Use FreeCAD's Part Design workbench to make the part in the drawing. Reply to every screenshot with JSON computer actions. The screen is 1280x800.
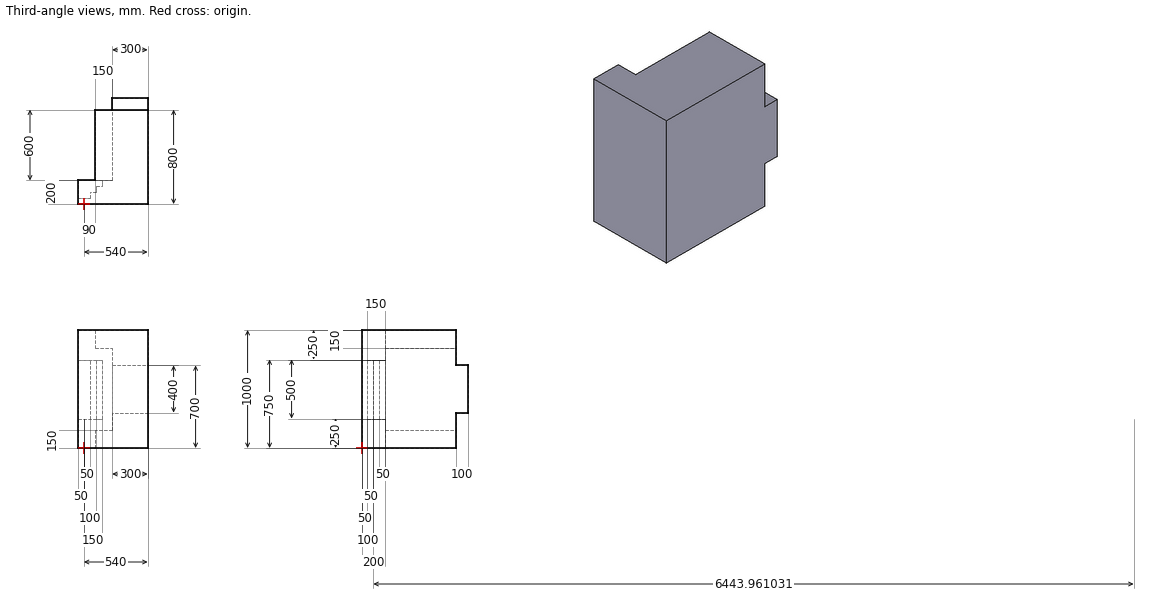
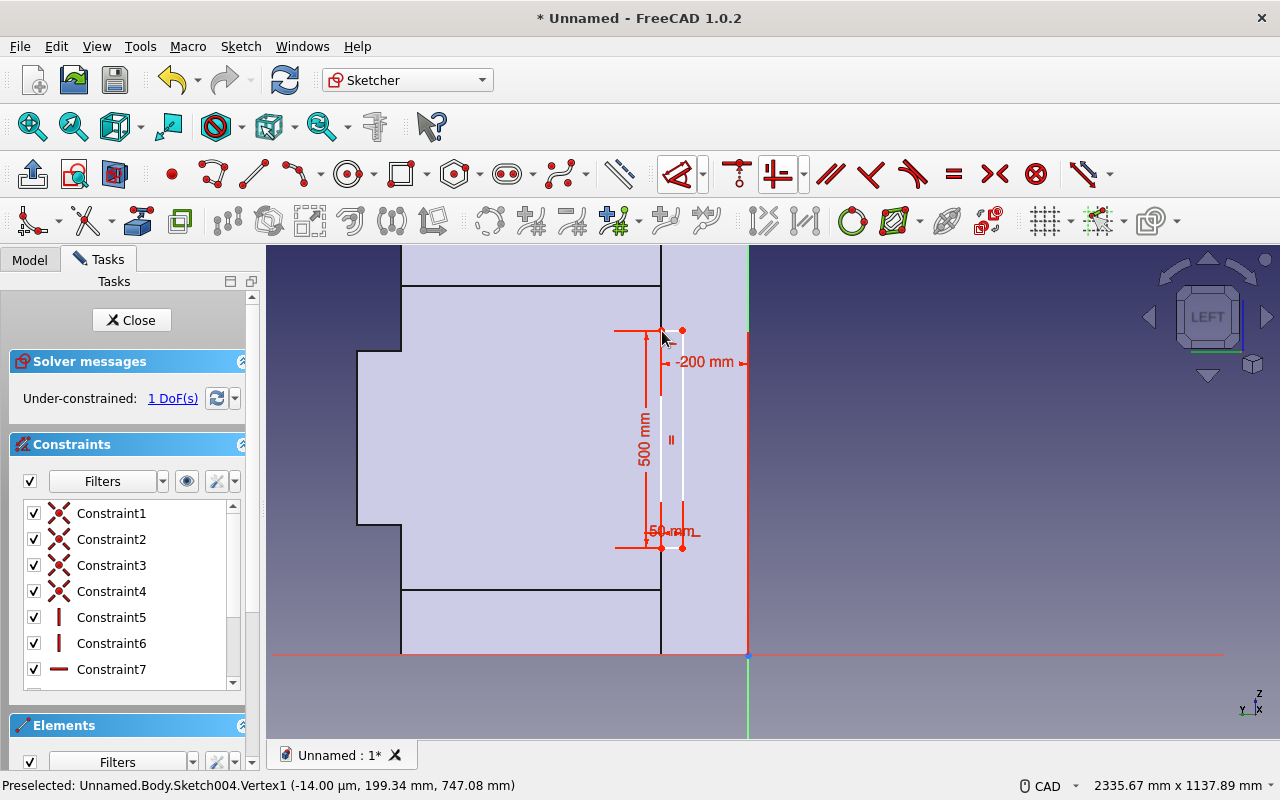
{"action": "left_click", "coordinate": [661, 331]}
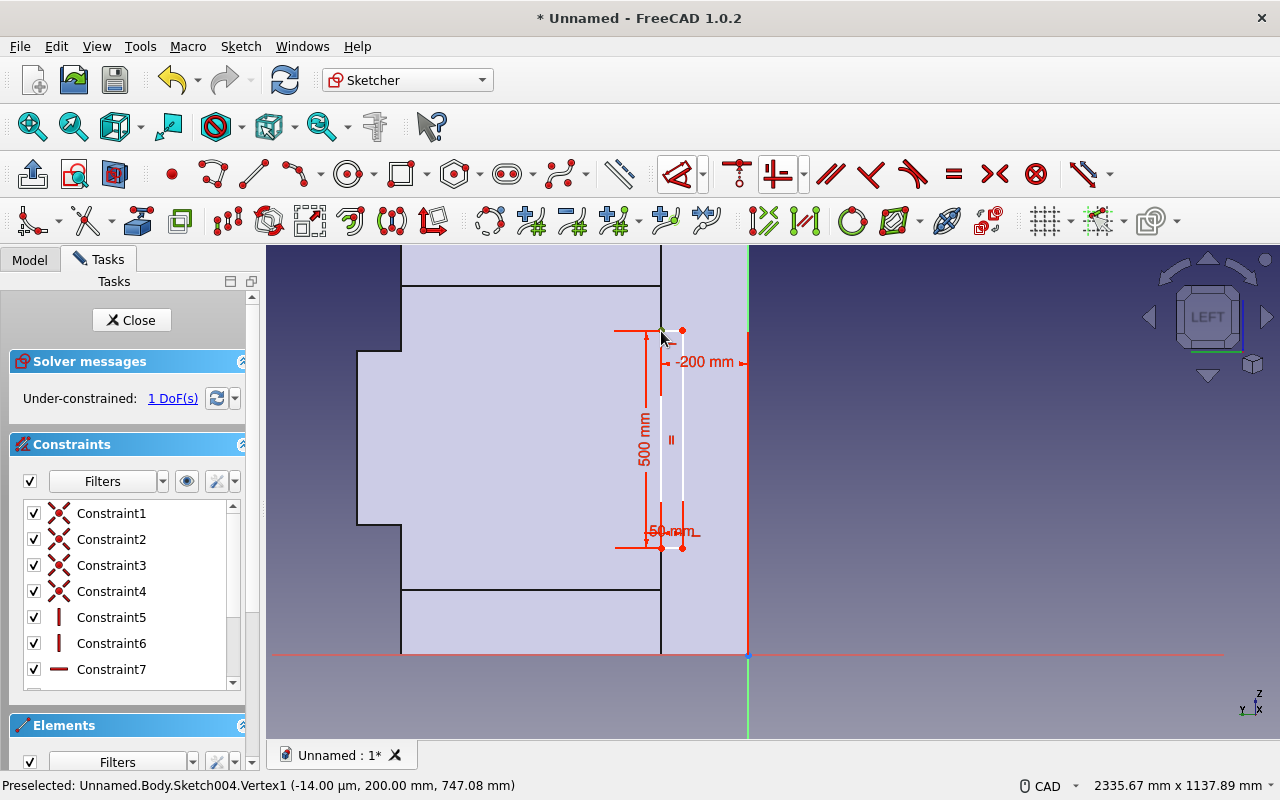
{"action": "key", "text": "i"}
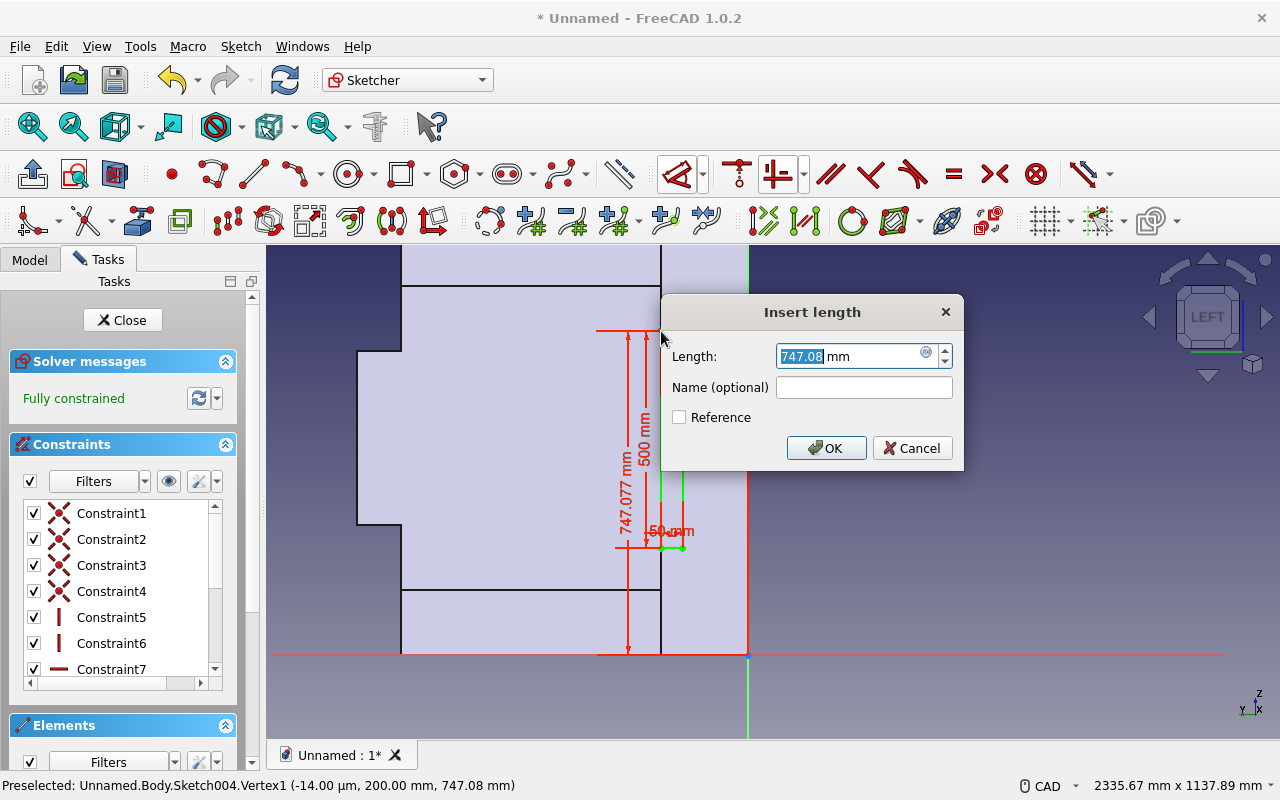
{"action": "type", "text": "750"}
{"action": "key", "text": "Return"}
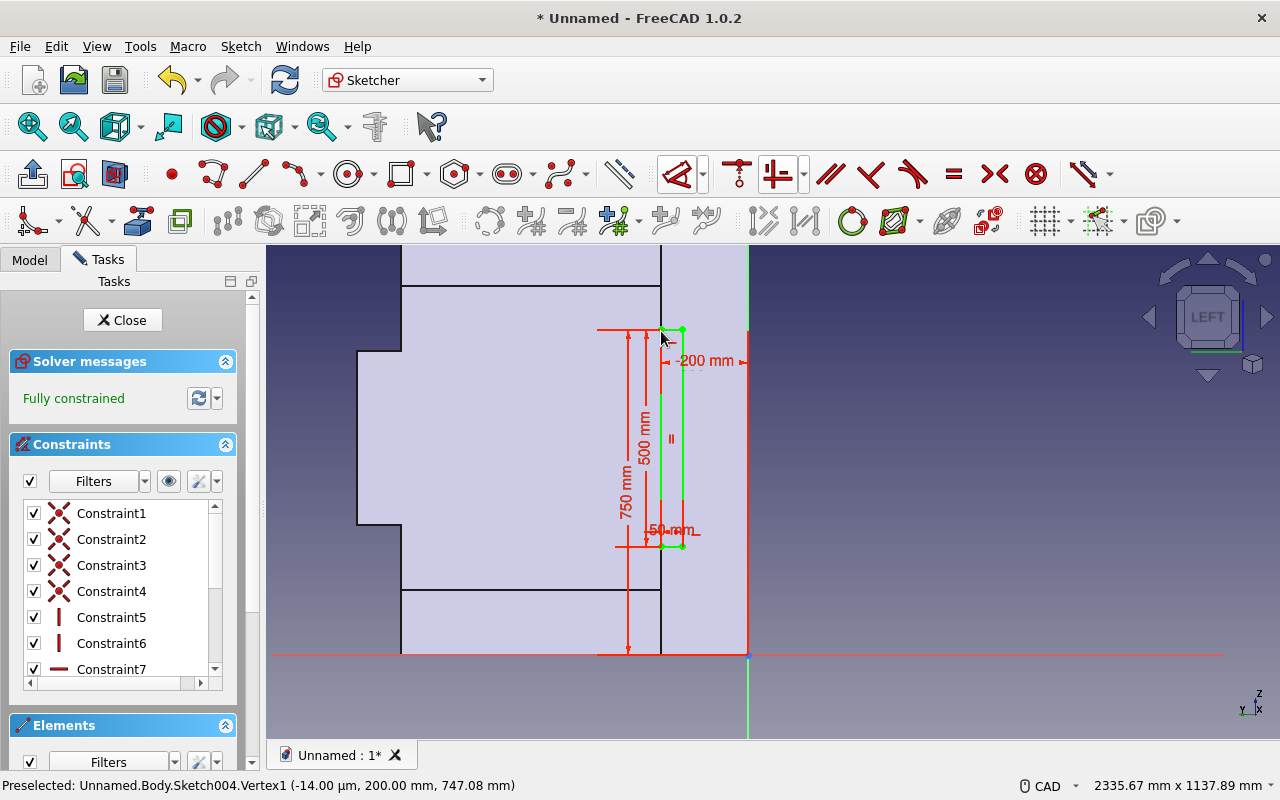
{"action": "left_click", "coordinate": [123, 320]}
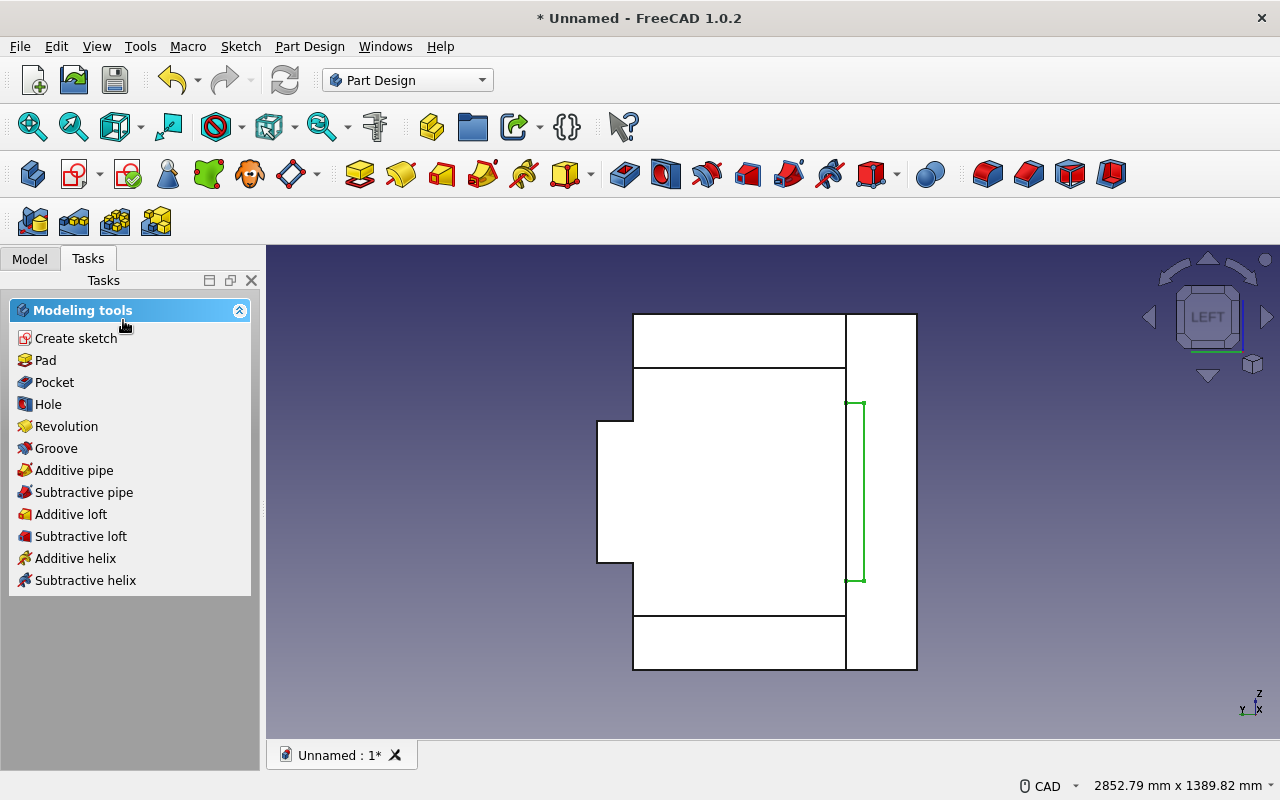
{"action": "left_click", "coordinate": [625, 174]}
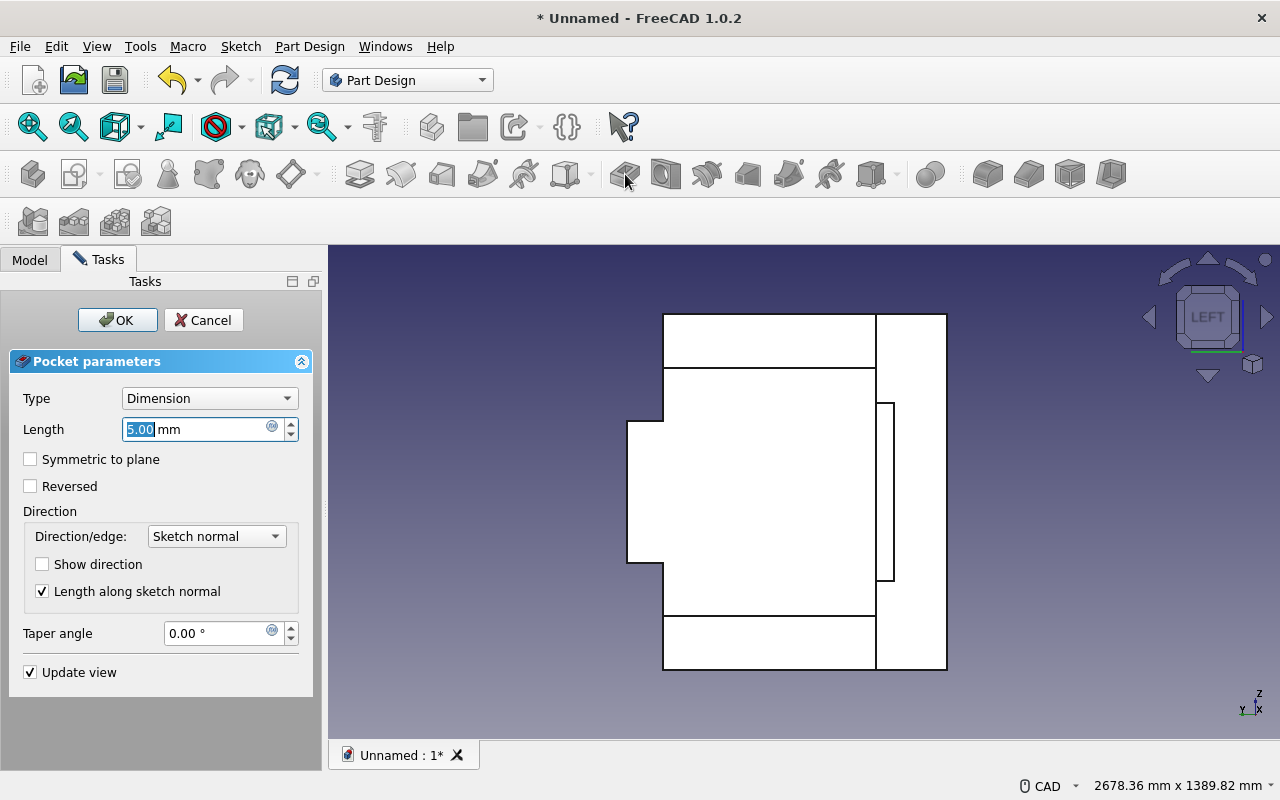
{"action": "type", "text": "150"}
{"action": "key", "text": "Tab"}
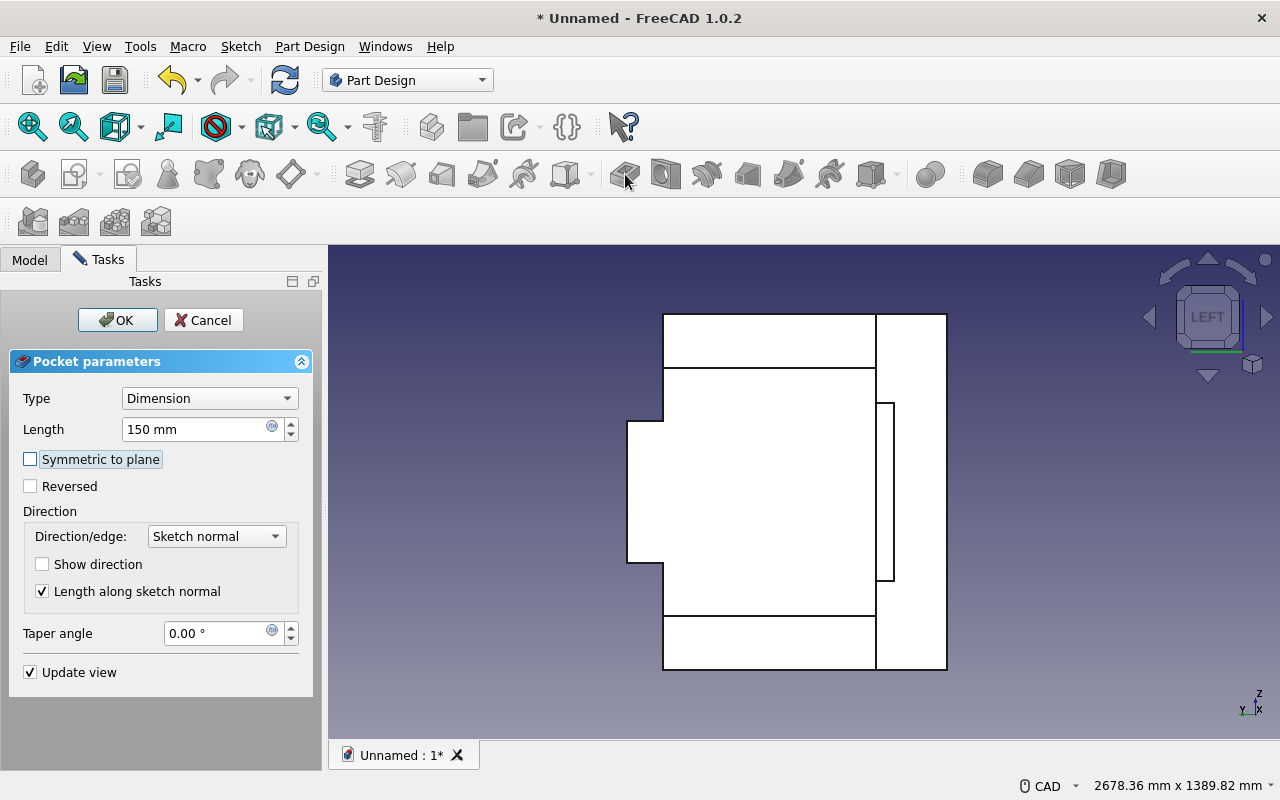
{"action": "left_click", "coordinate": [118, 320]}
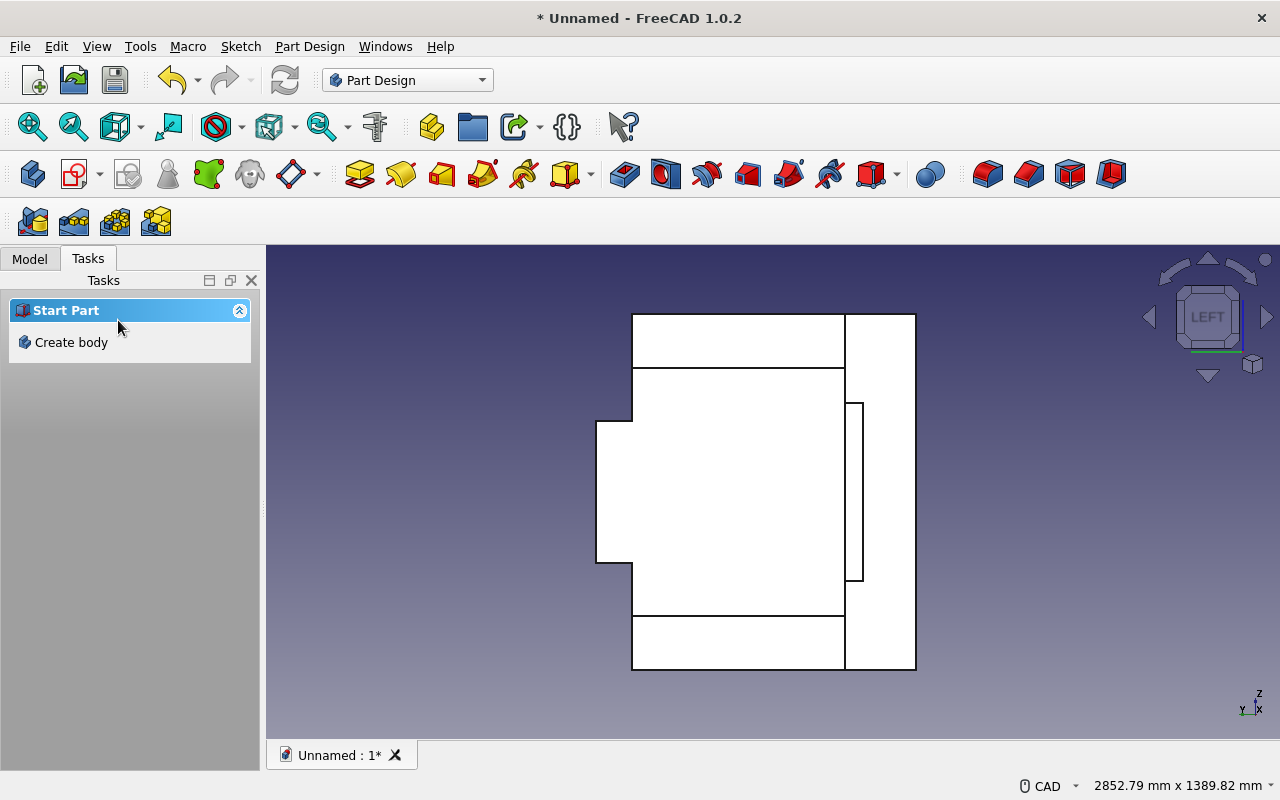
{"action": "left_click", "coordinate": [74, 174]}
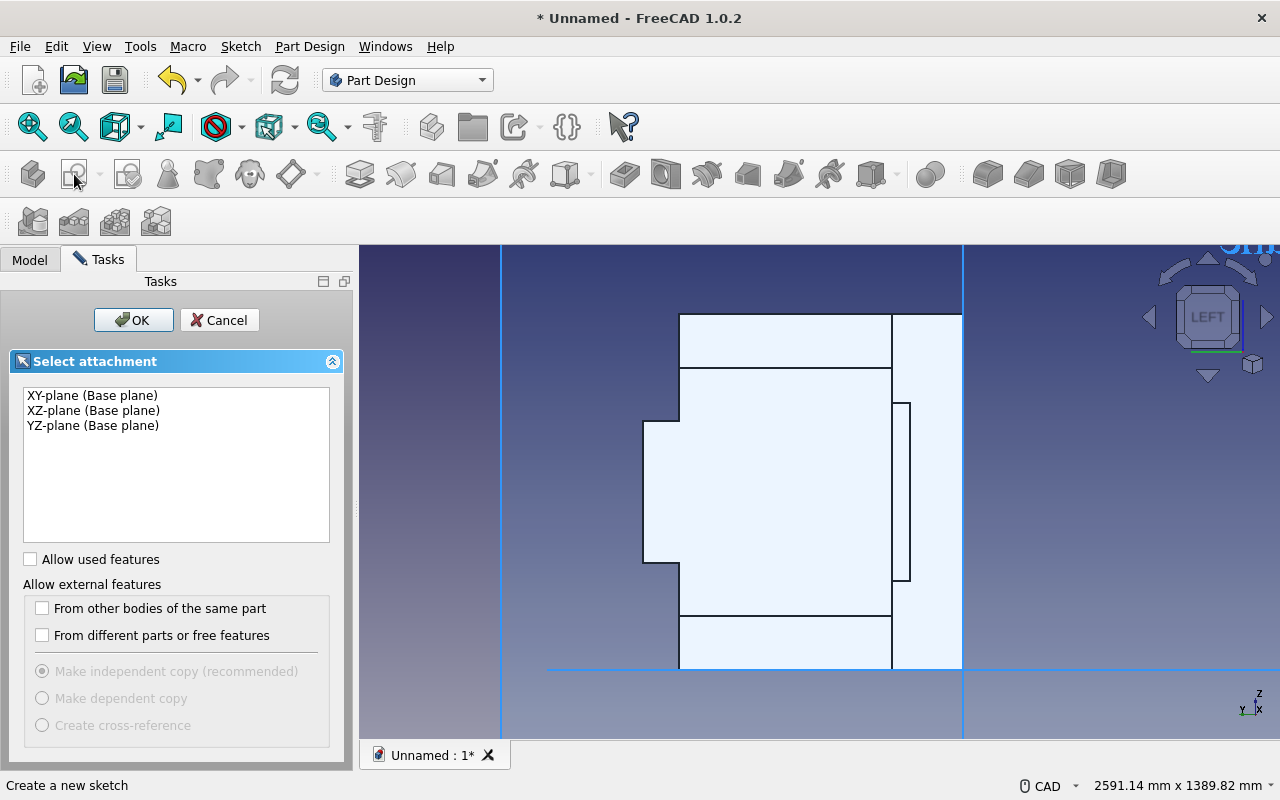
{"action": "left_click", "coordinate": [84, 426]}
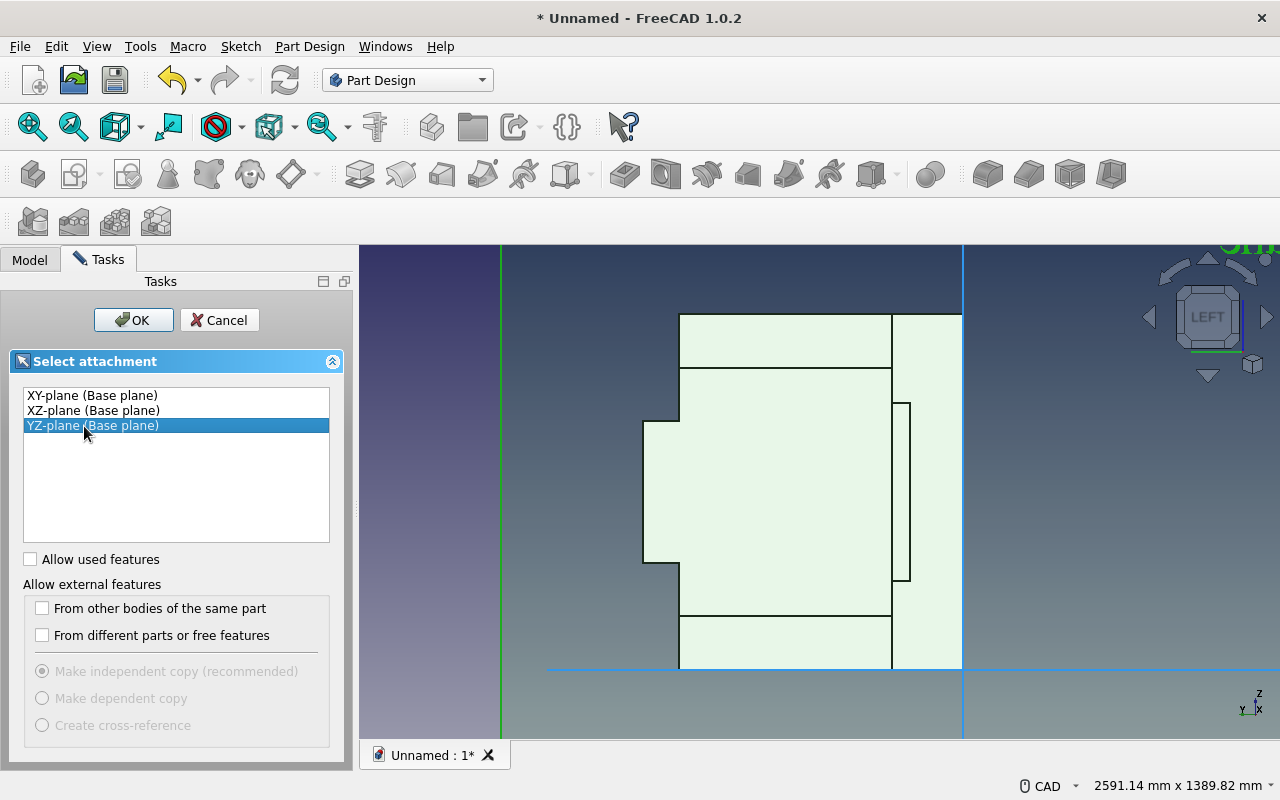
{"action": "left_click", "coordinate": [134, 320]}